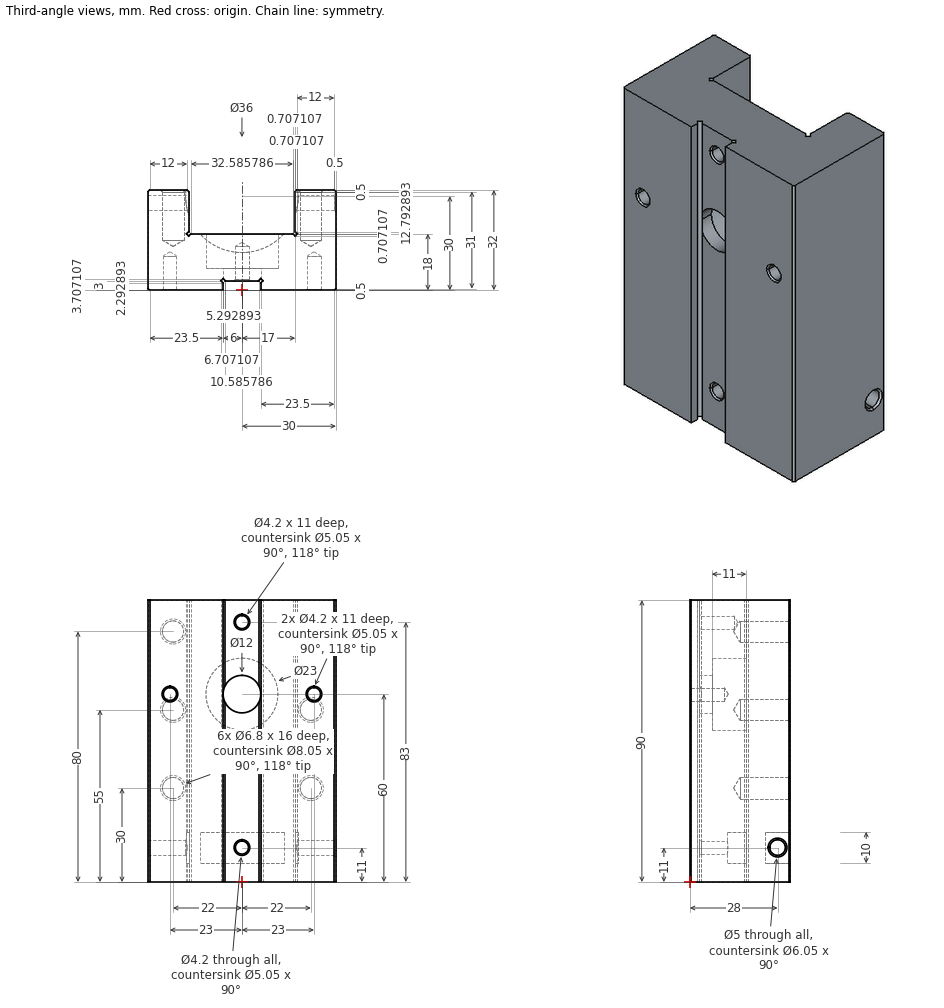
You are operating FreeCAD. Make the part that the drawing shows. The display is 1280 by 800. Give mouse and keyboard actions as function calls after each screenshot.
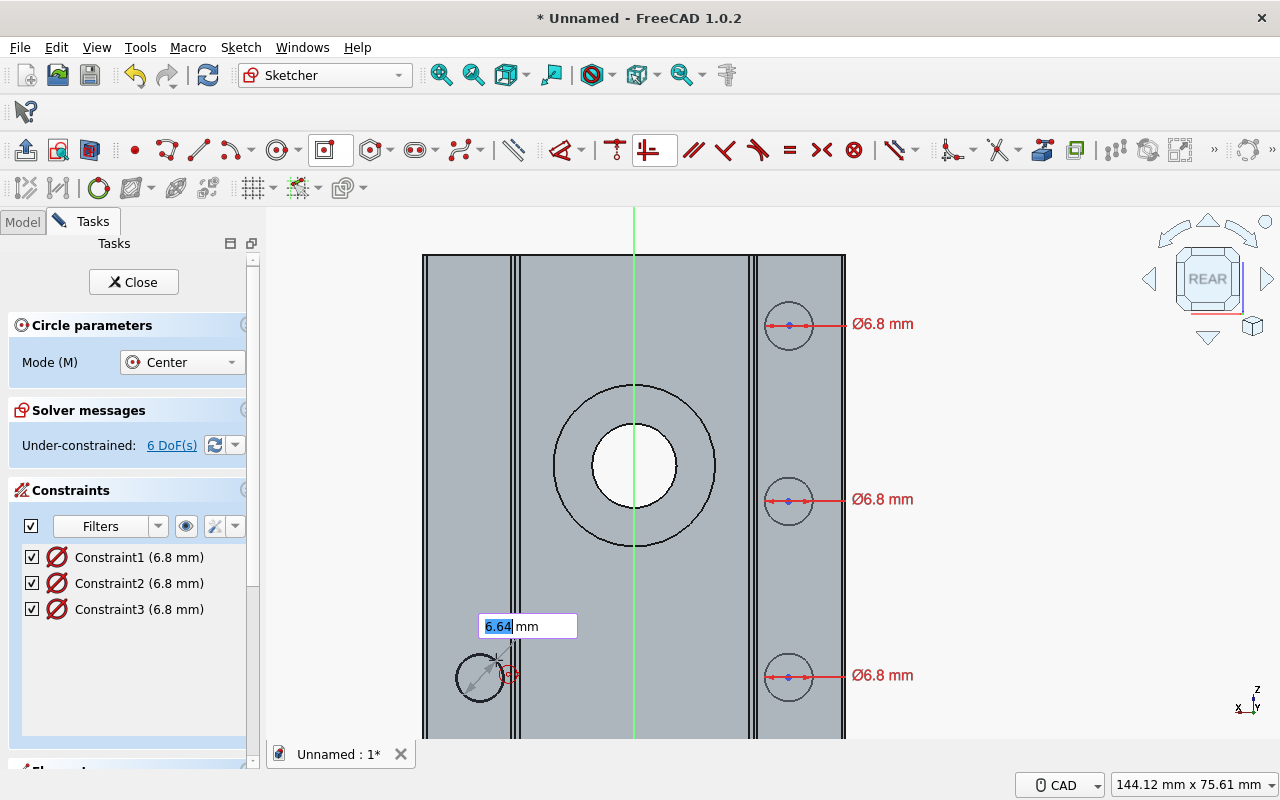
text(6.8)
key(Return)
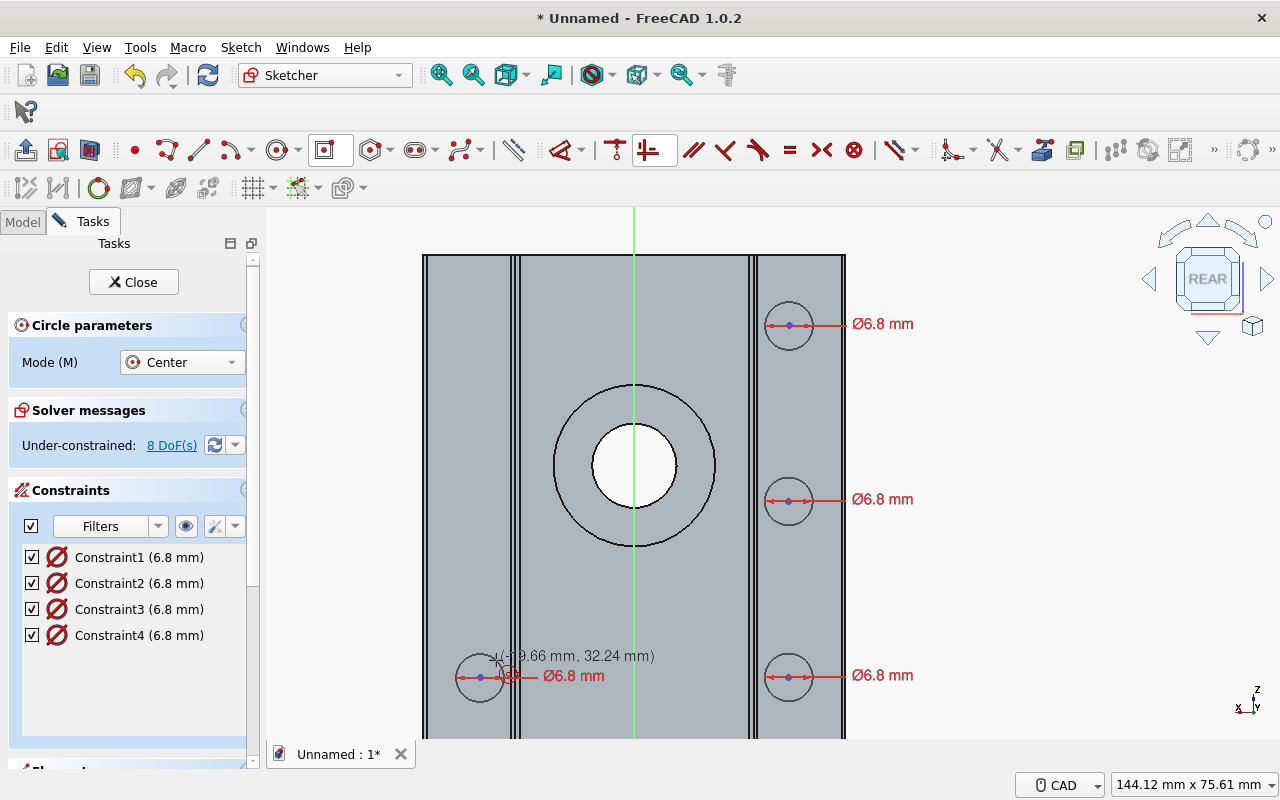
click(480, 501)
move(496, 484)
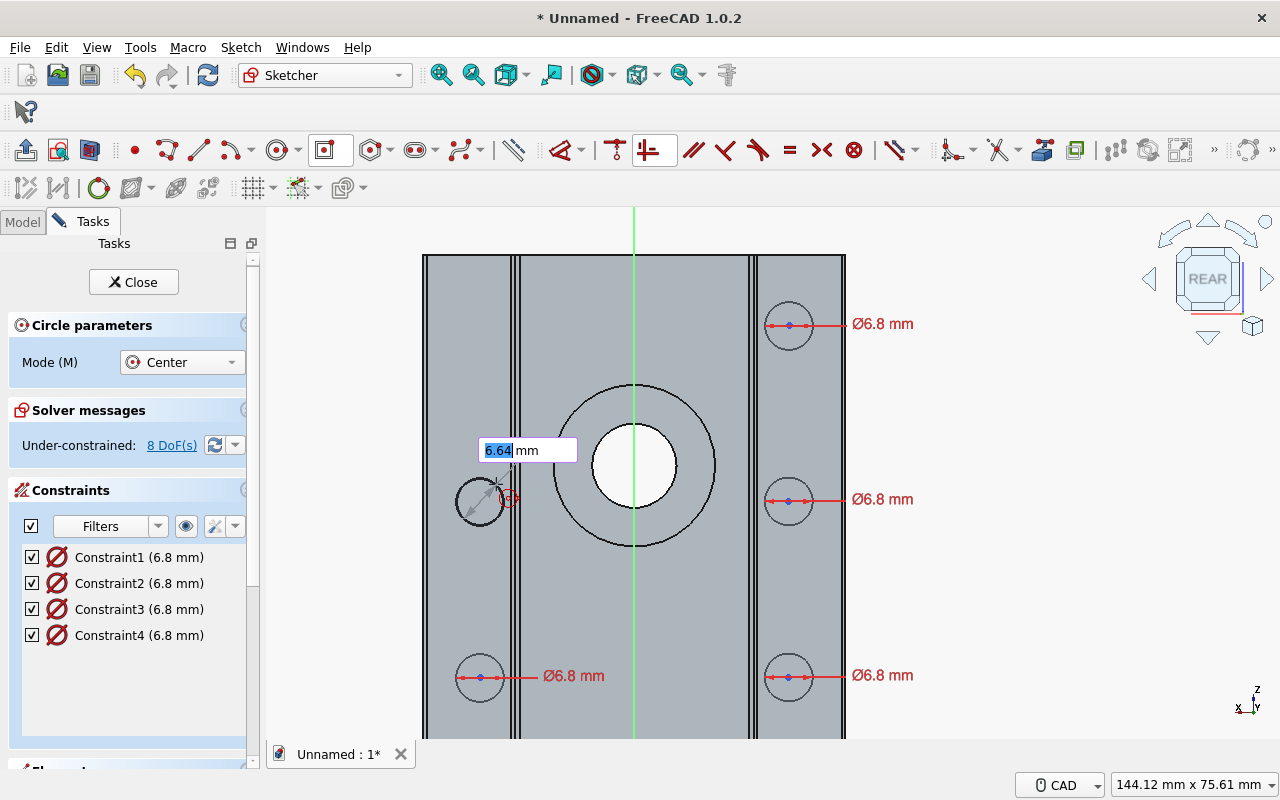
text(6.8)
key(Return)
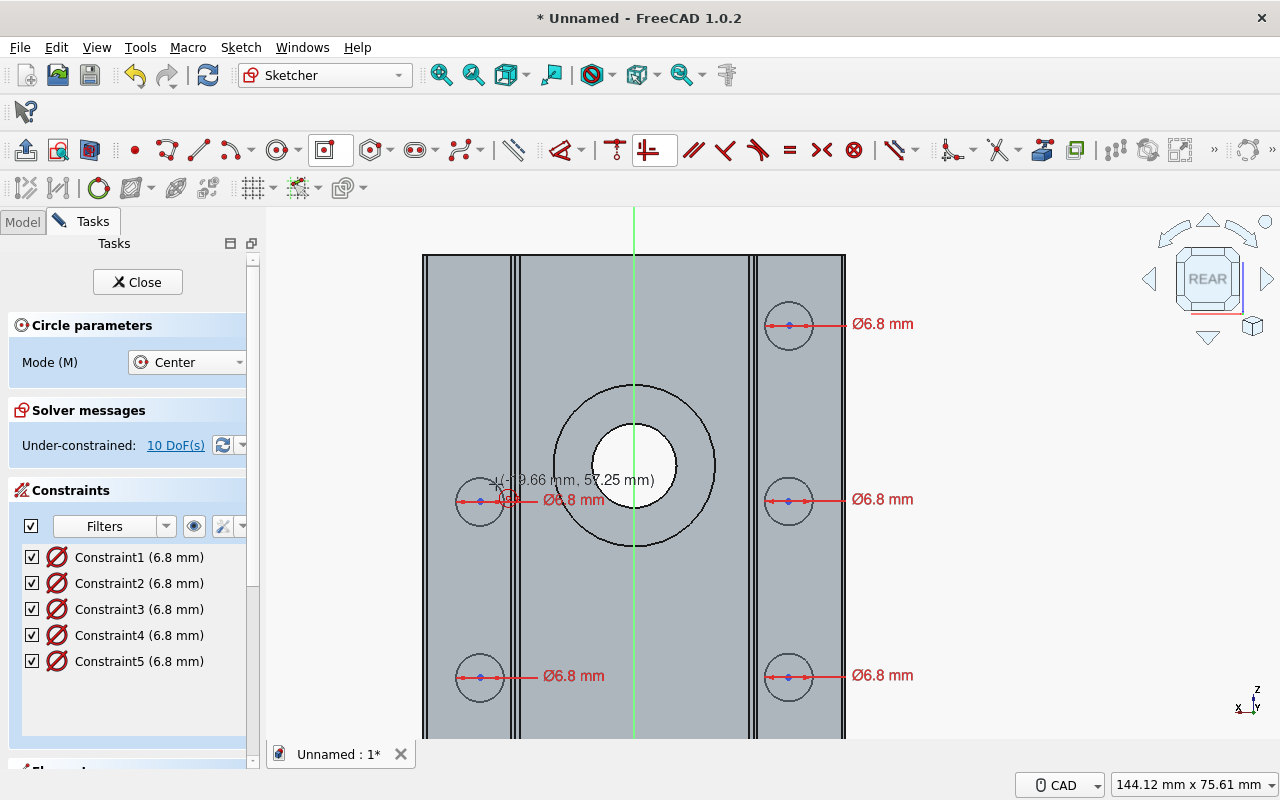
click(480, 325)
move(496, 308)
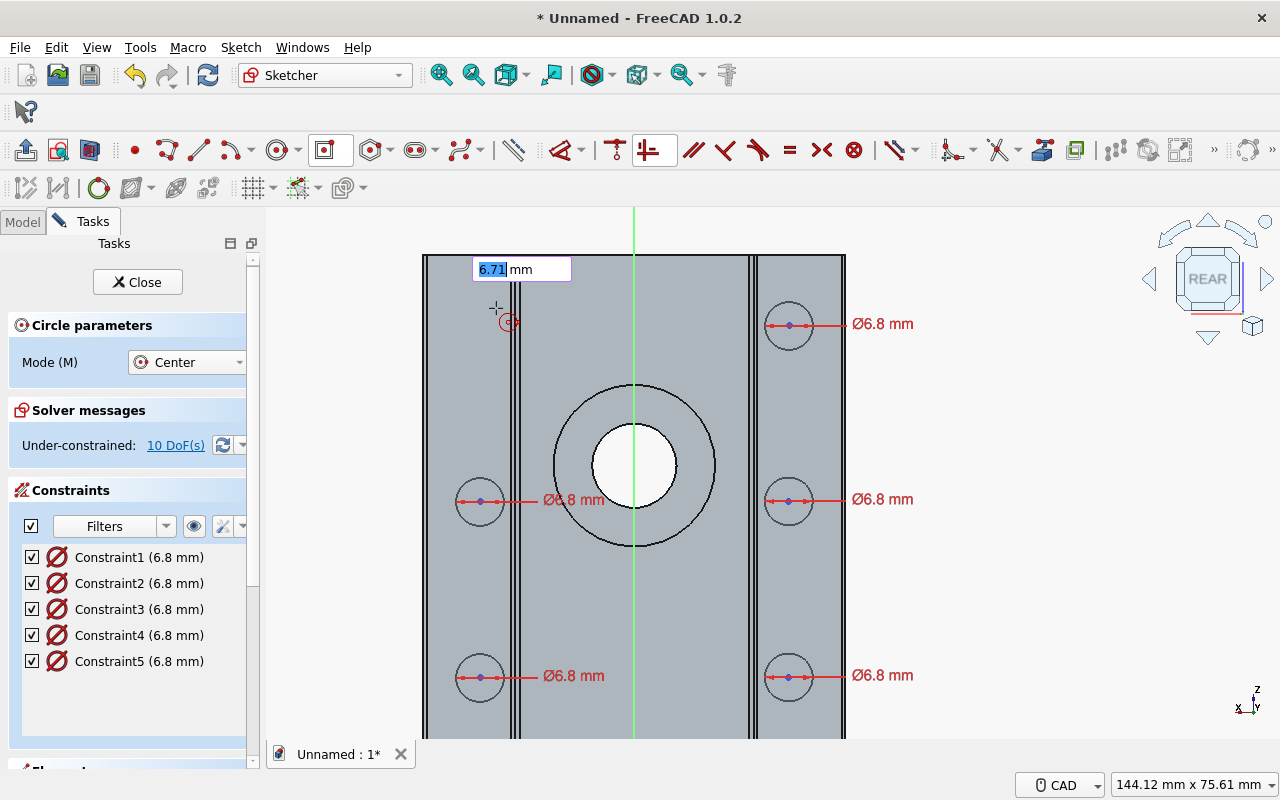
text(6.8)
key(Return)
key(Escape)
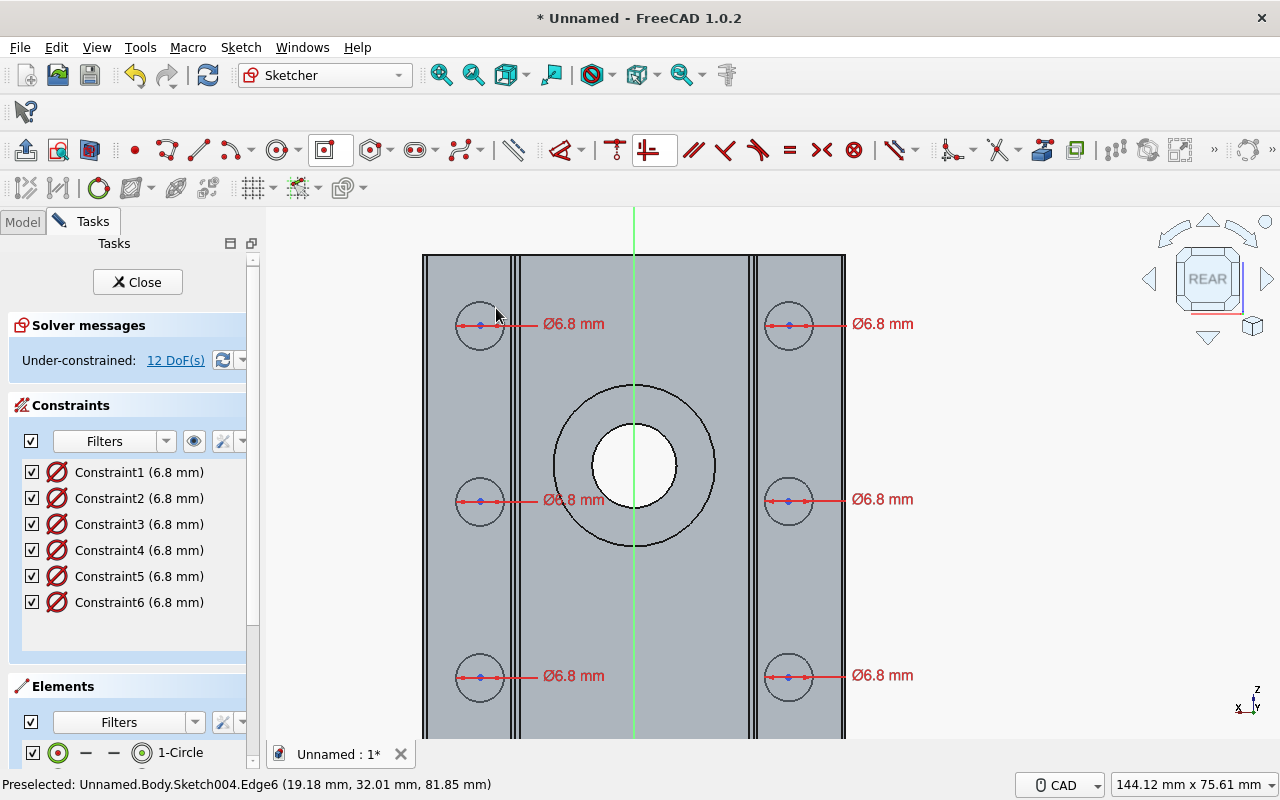
click(789, 677)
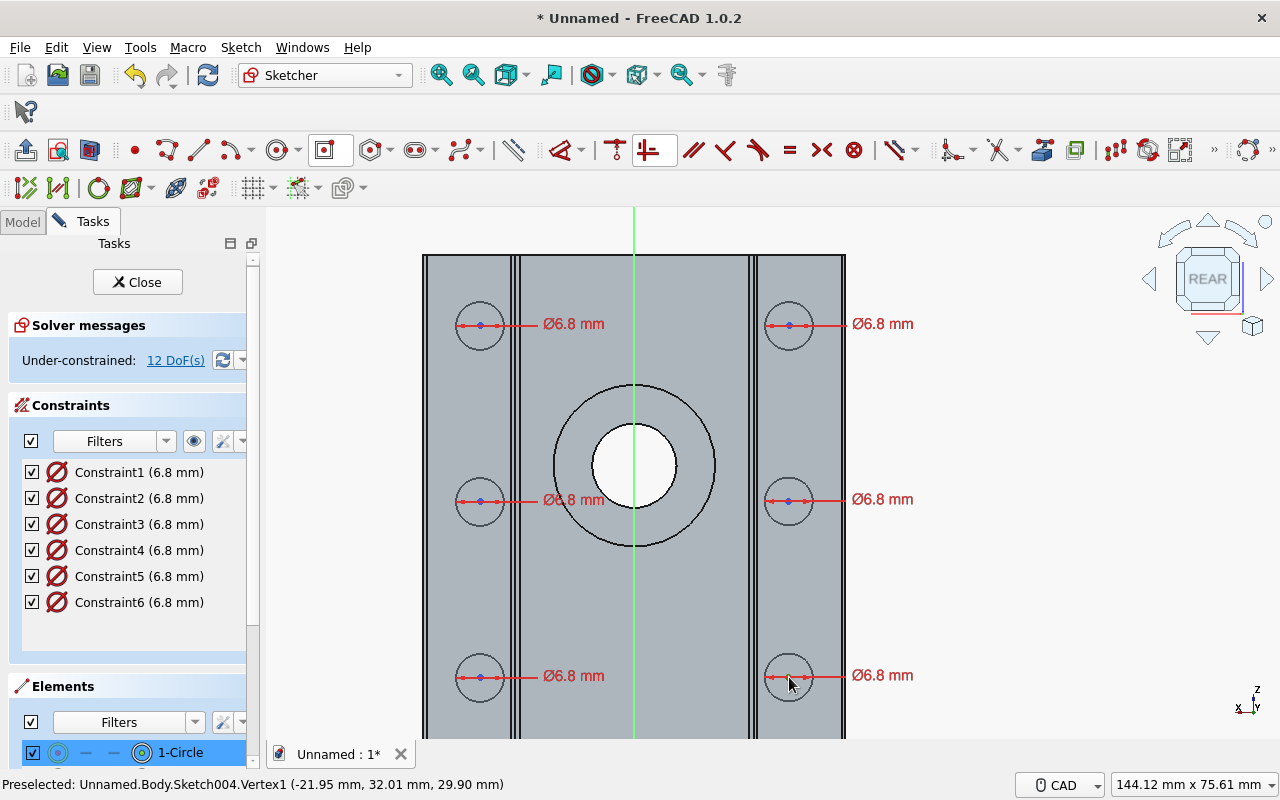
click(789, 501)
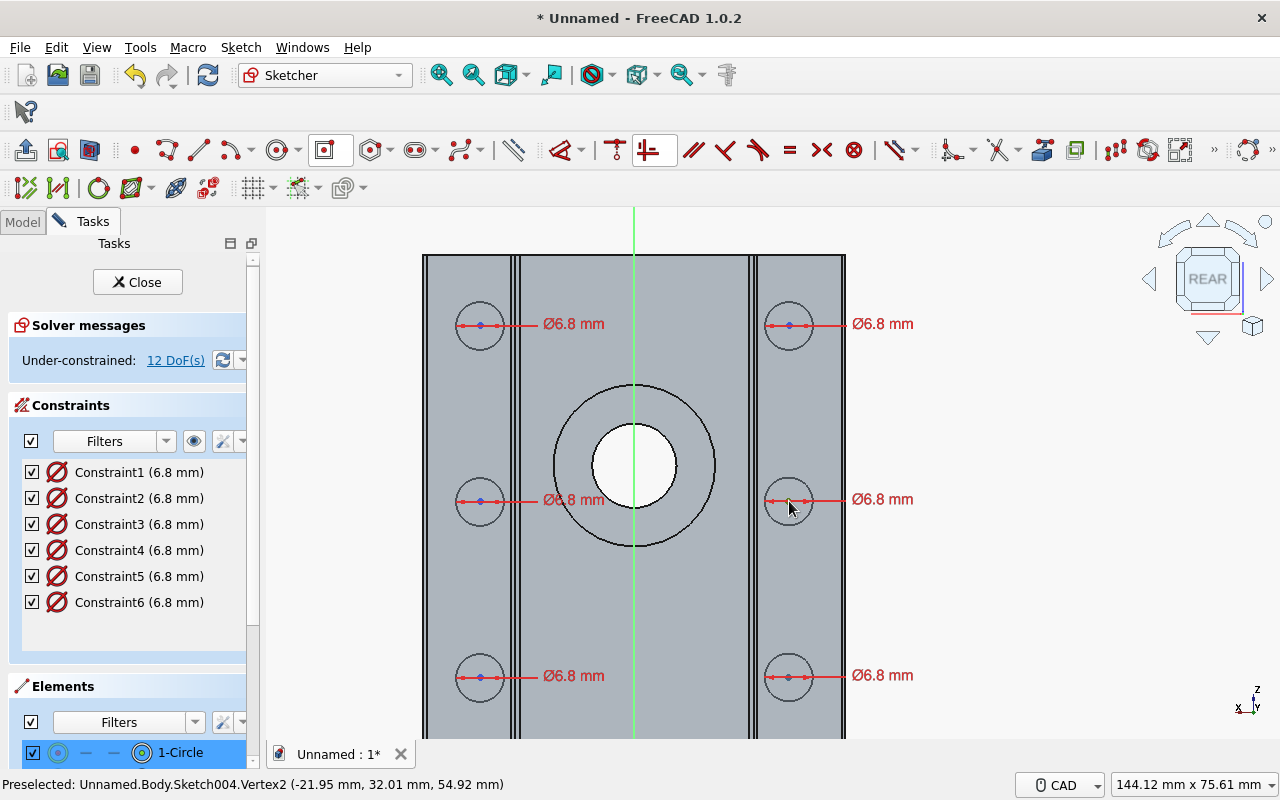
click(672, 150)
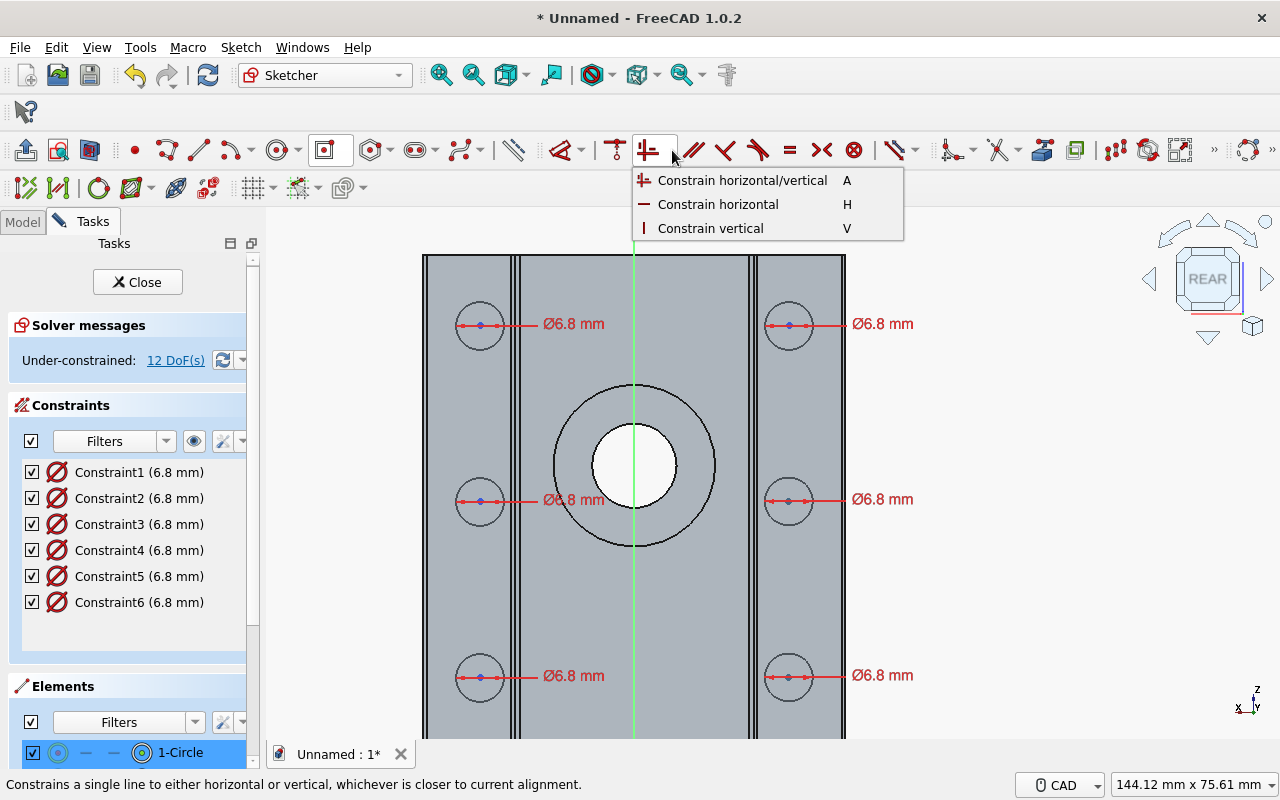
click(768, 228)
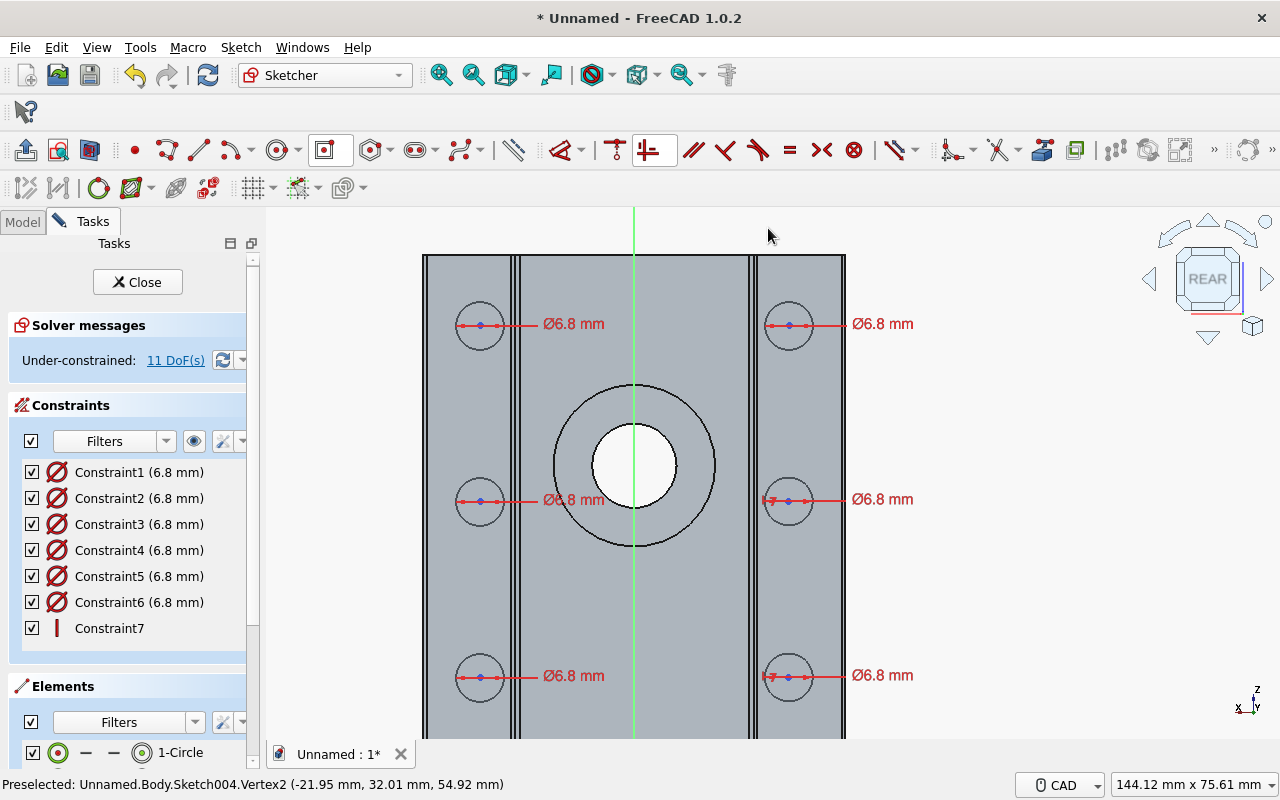
click(789, 501)